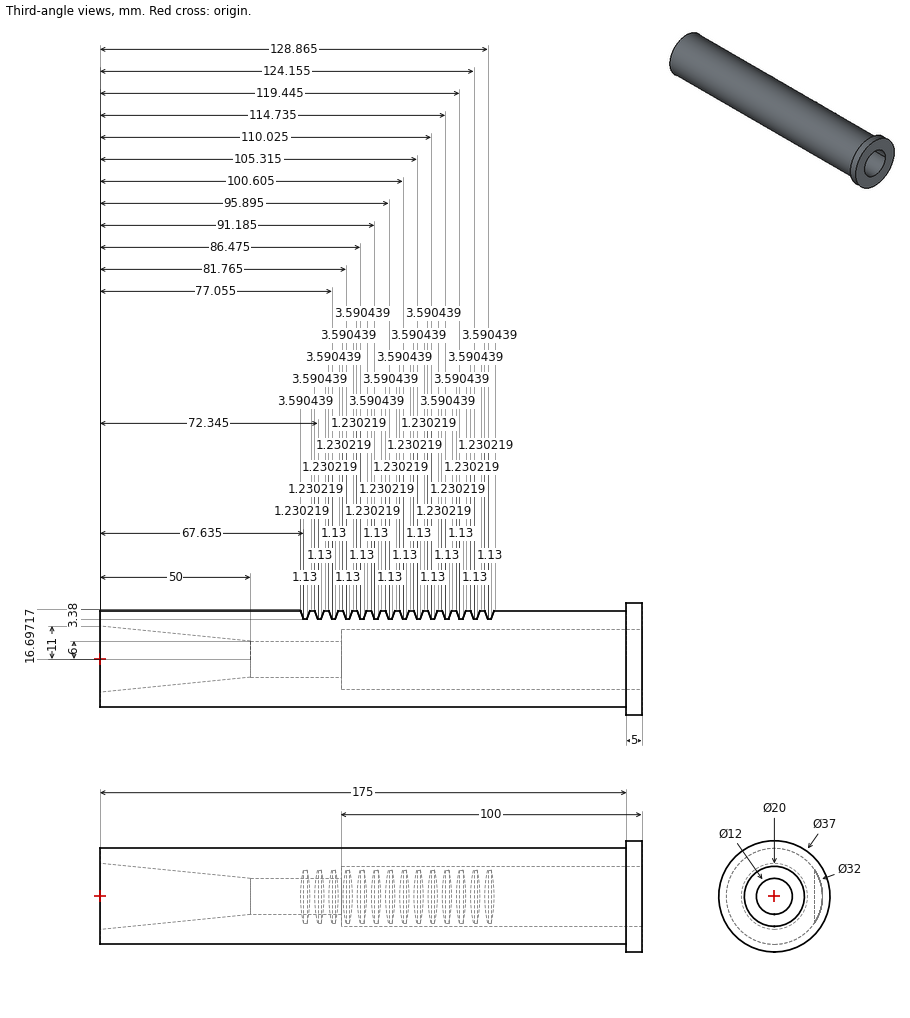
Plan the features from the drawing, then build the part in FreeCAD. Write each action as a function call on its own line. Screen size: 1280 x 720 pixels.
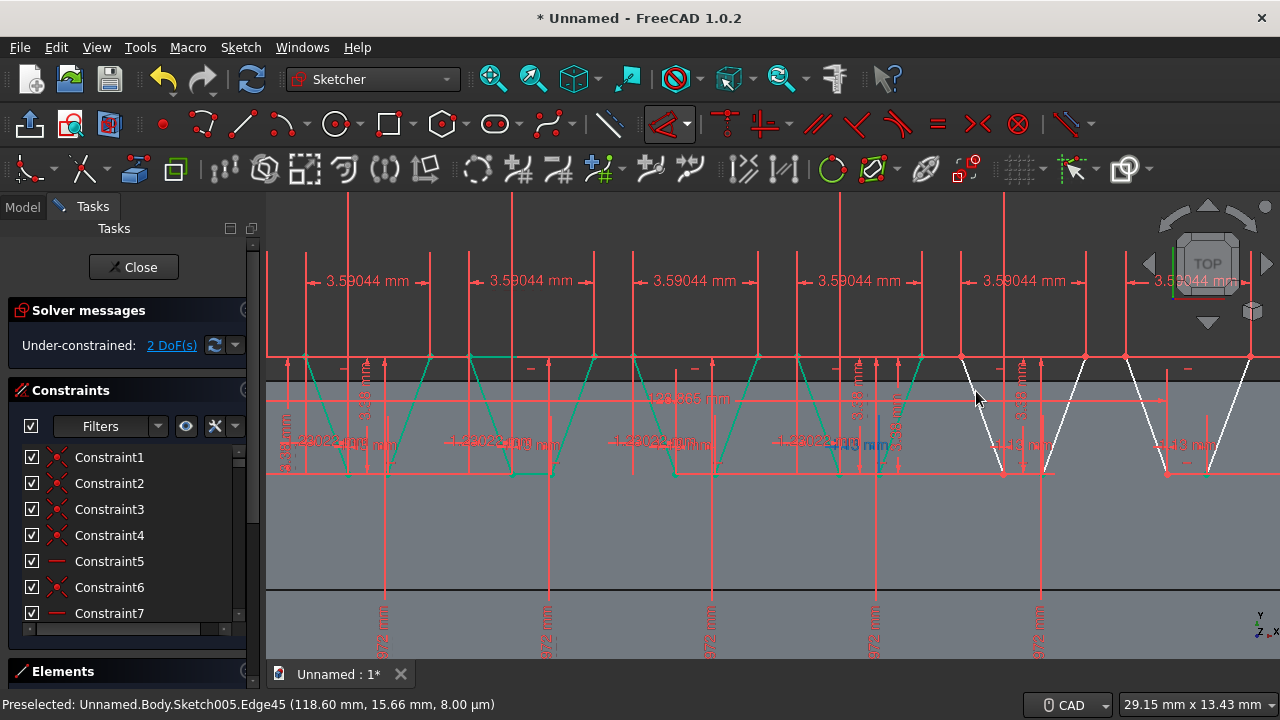
click(974, 392)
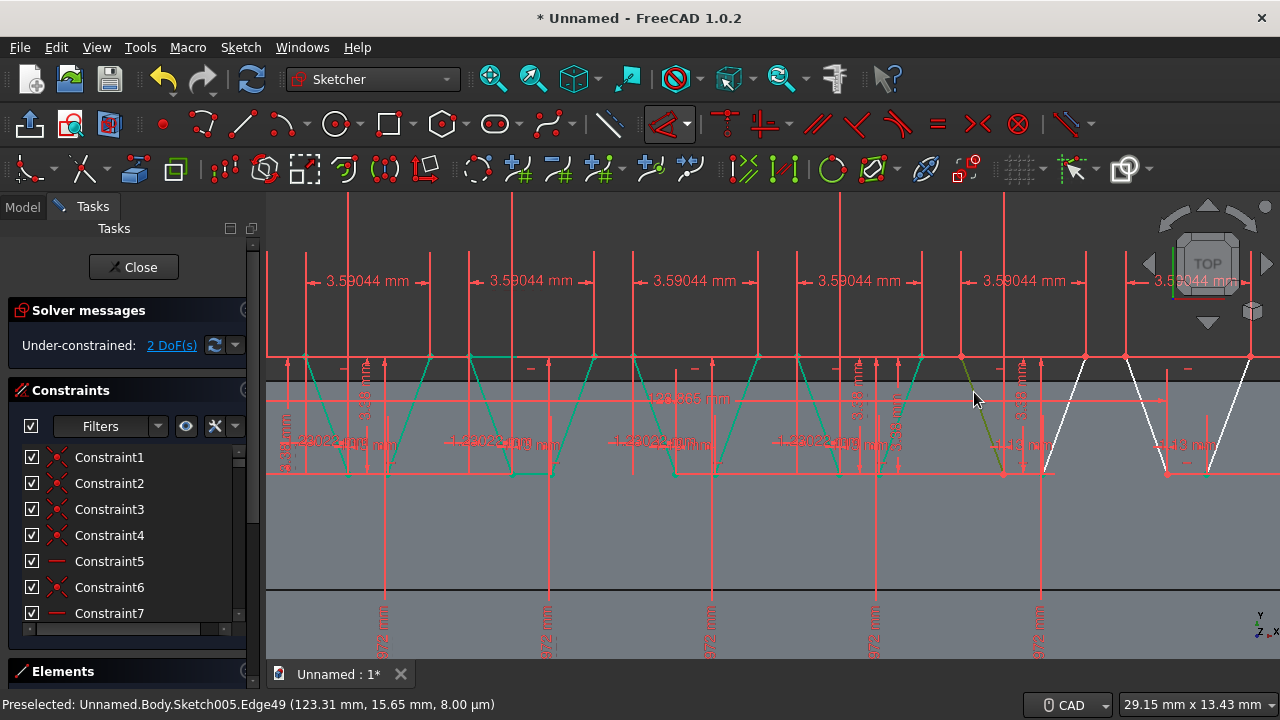
key(l)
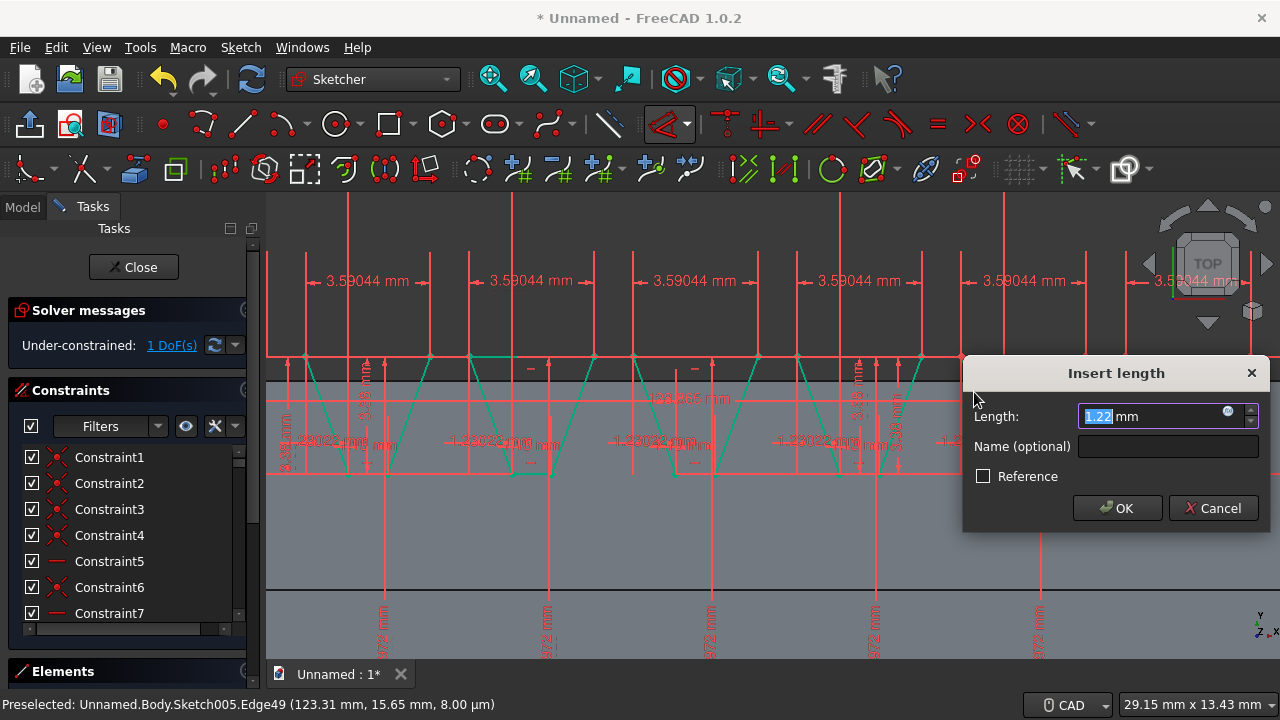
text(1.230219)
key(Return)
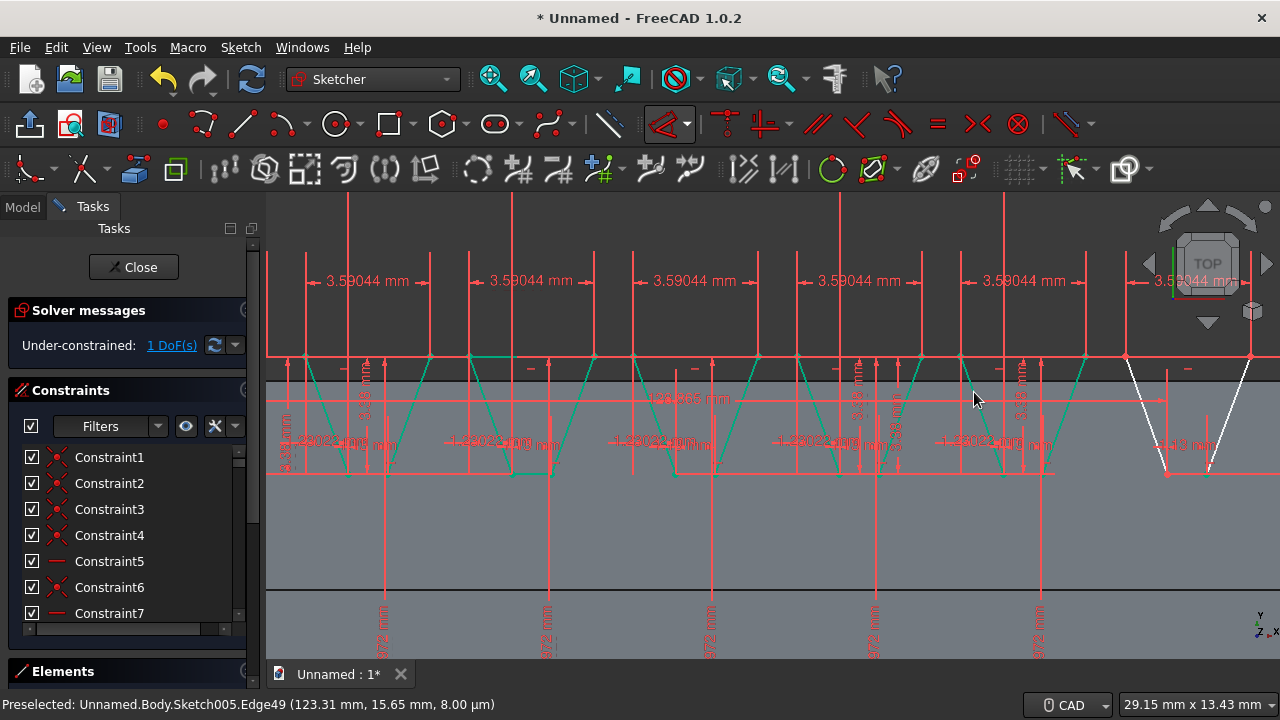
scroll(976, 391, down, 10)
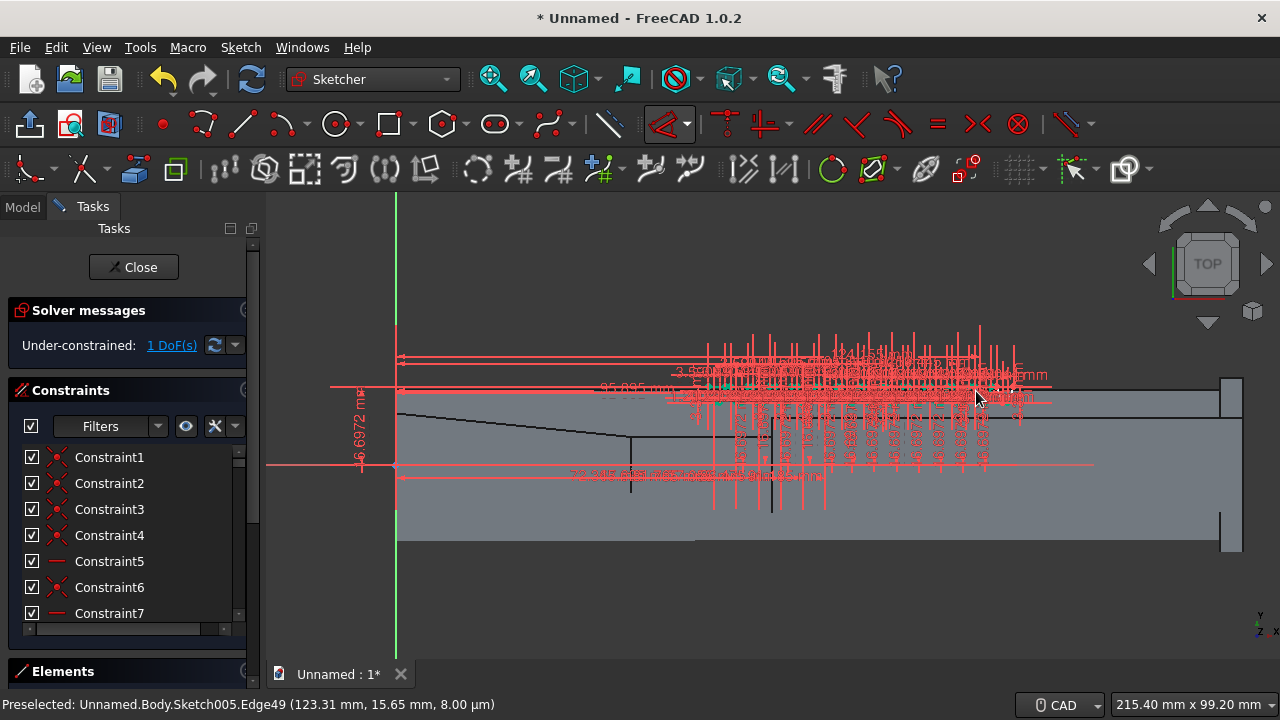
scroll(999, 391, up, 10)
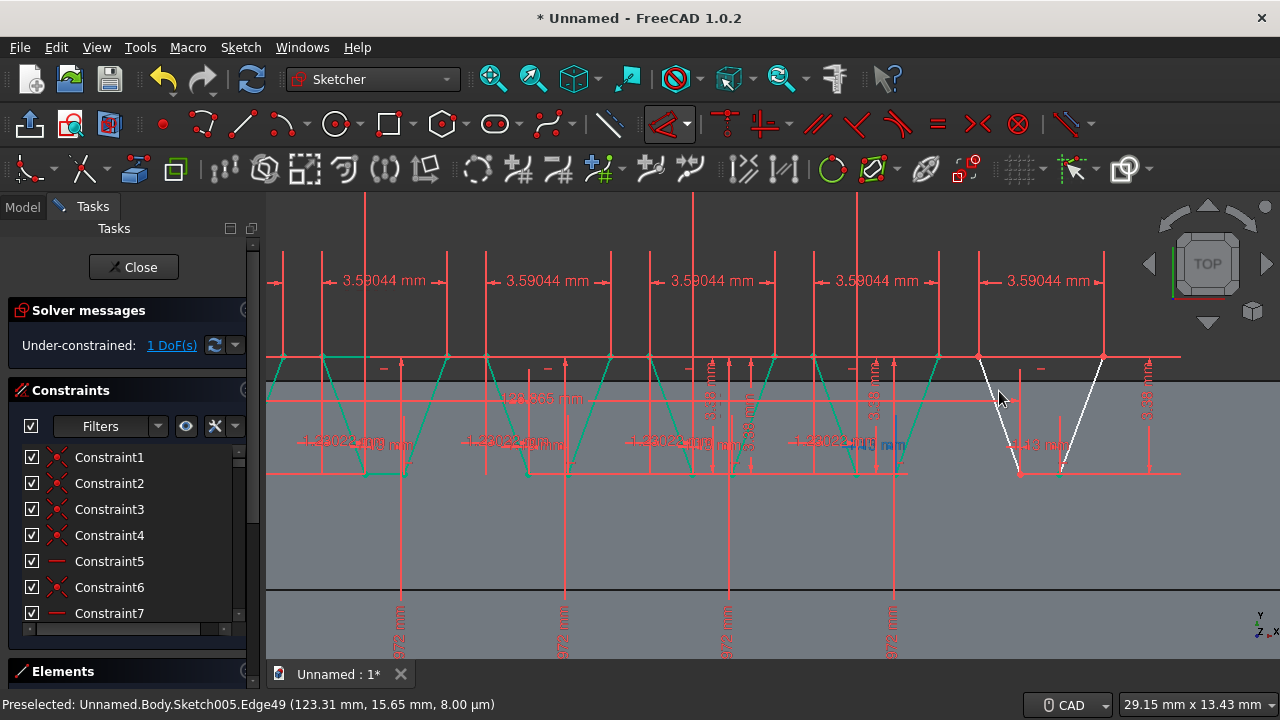
click(991, 392)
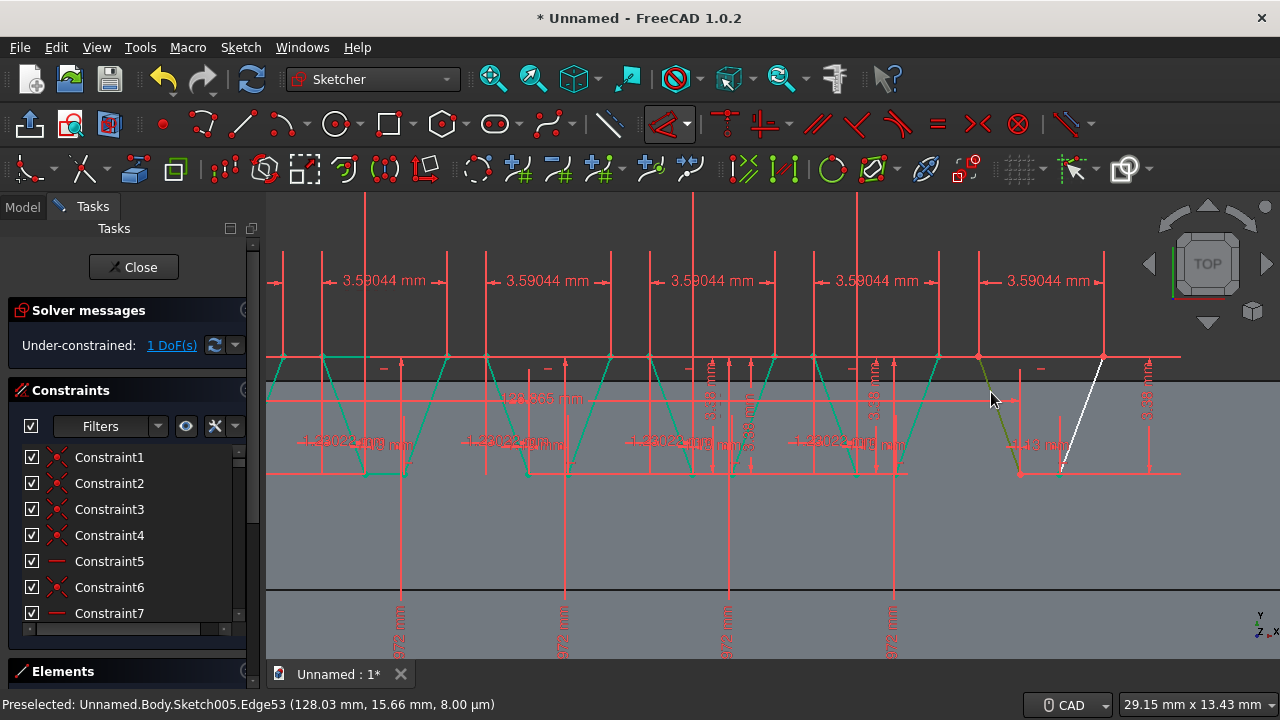
key(l)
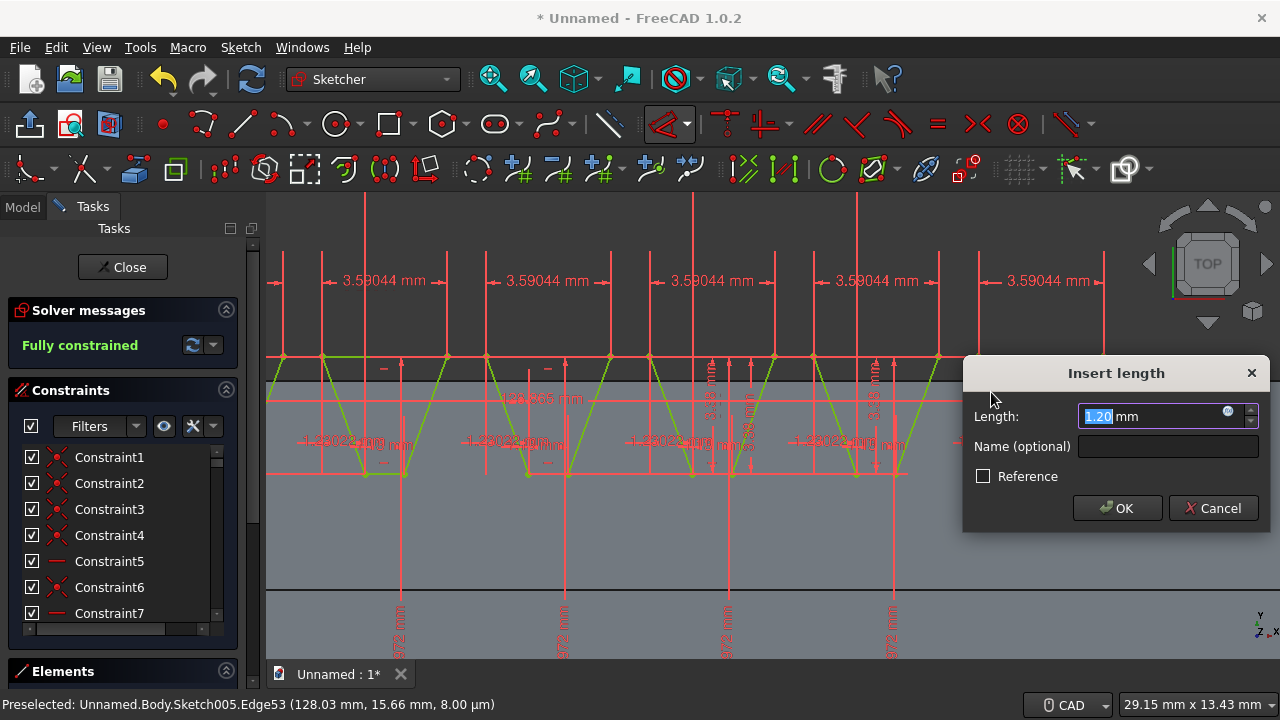
text(1.230219)
key(Return)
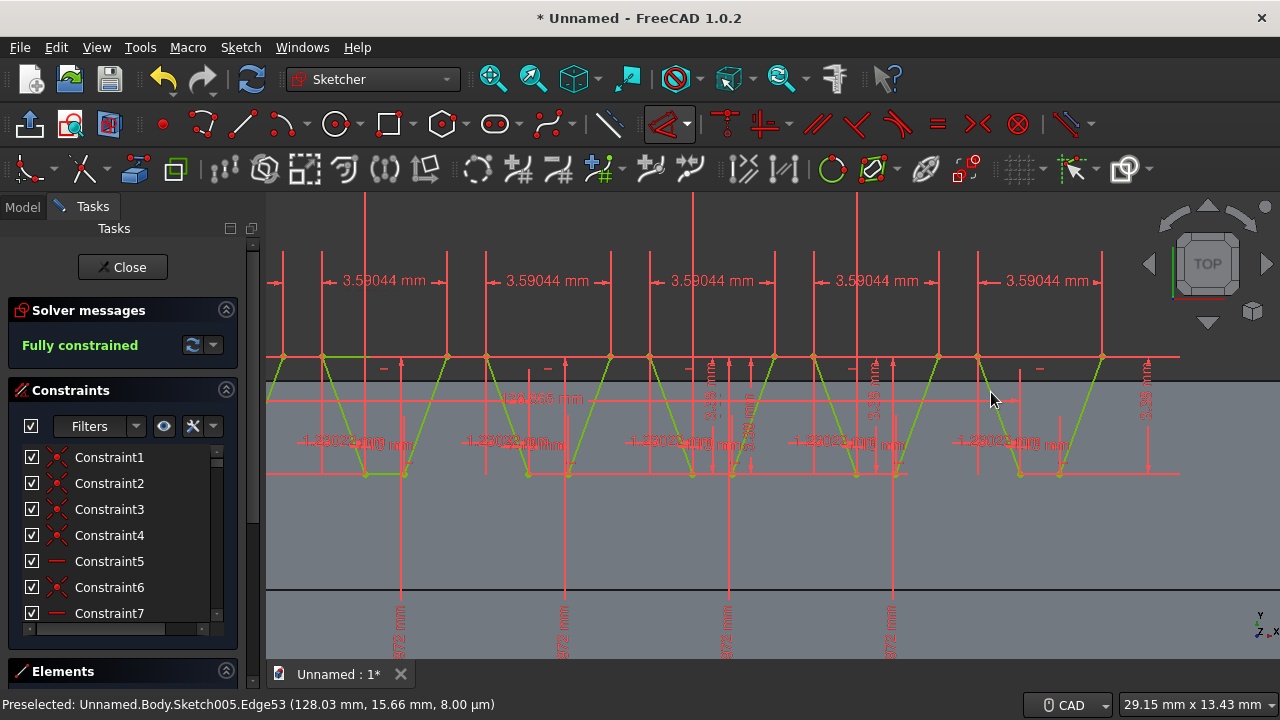
click(123, 267)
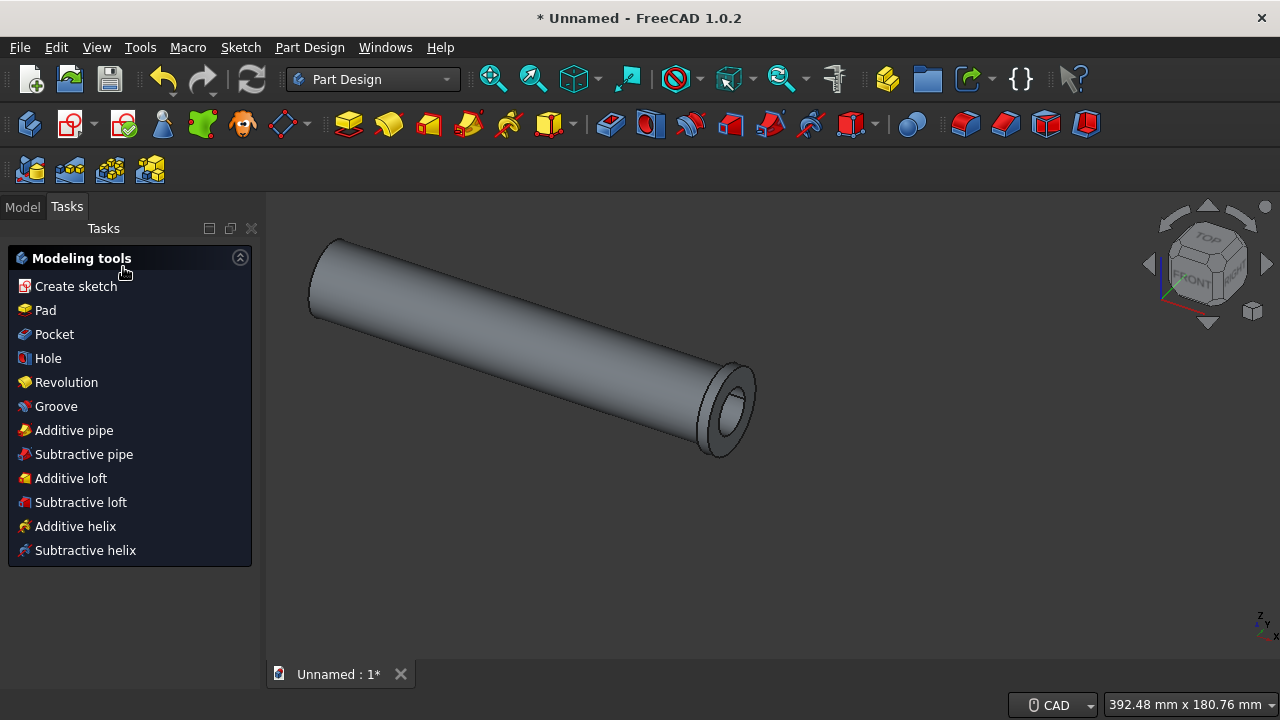
click(612, 124)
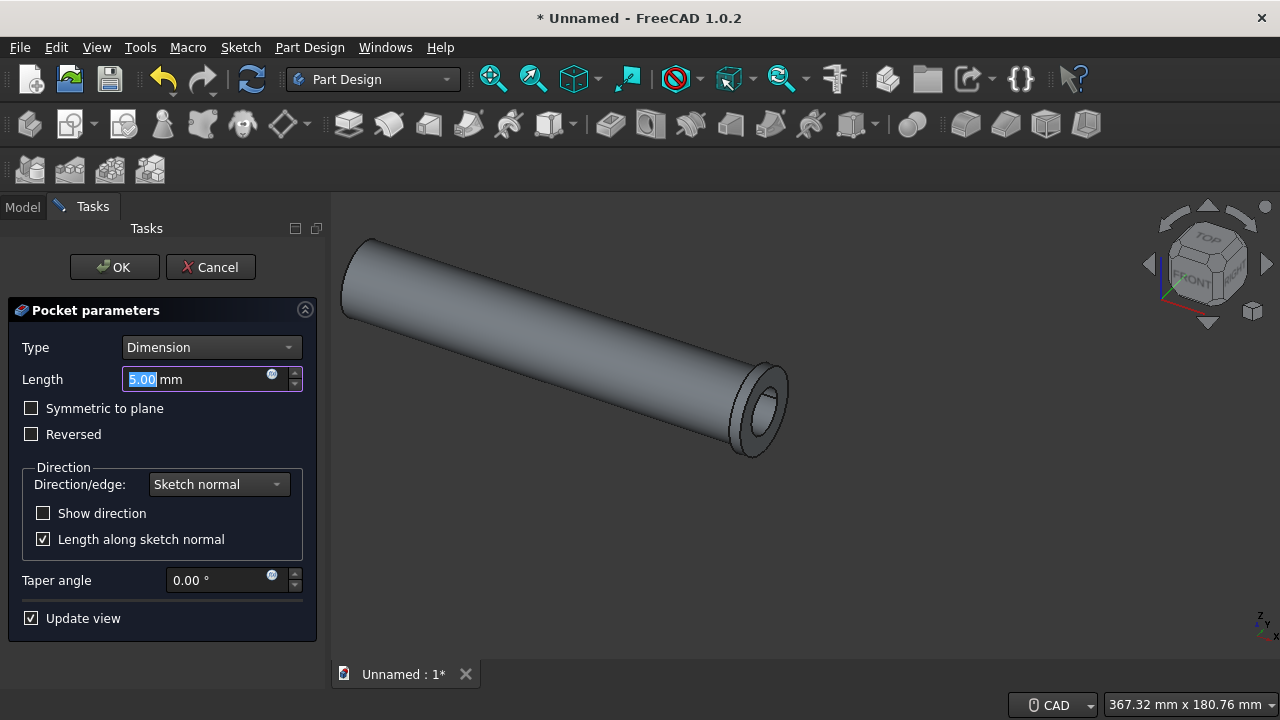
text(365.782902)
key(Tab)